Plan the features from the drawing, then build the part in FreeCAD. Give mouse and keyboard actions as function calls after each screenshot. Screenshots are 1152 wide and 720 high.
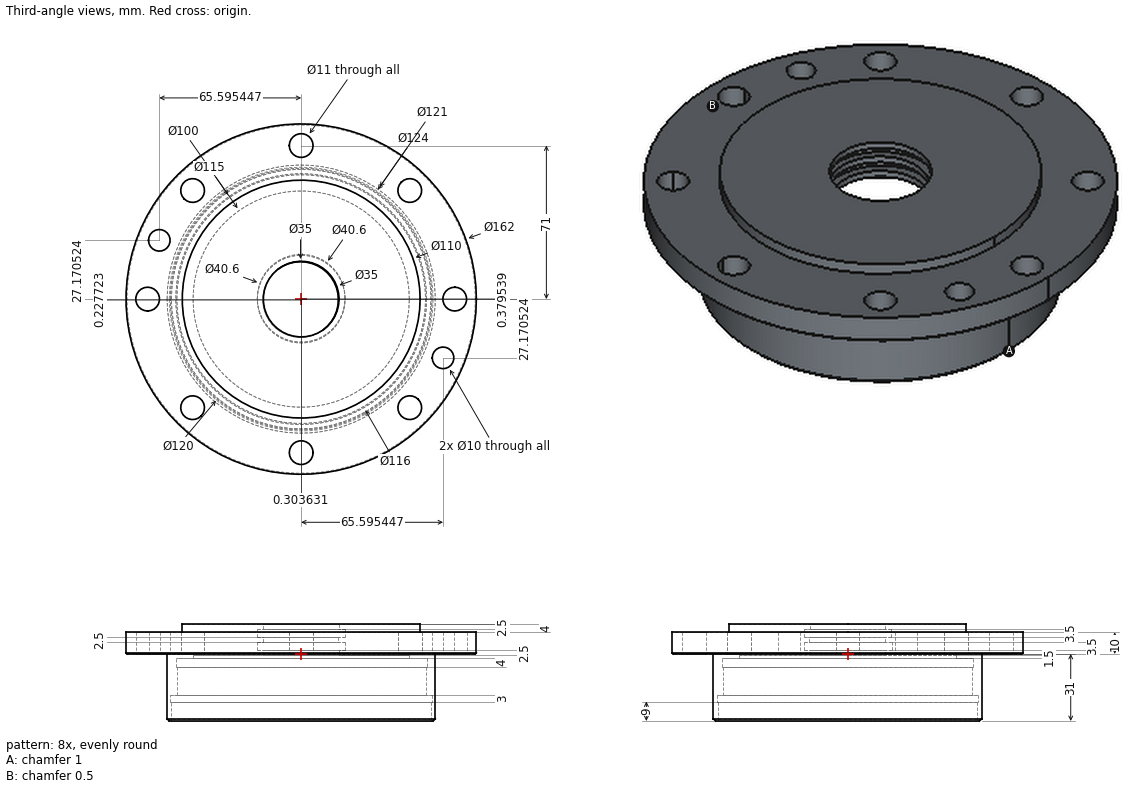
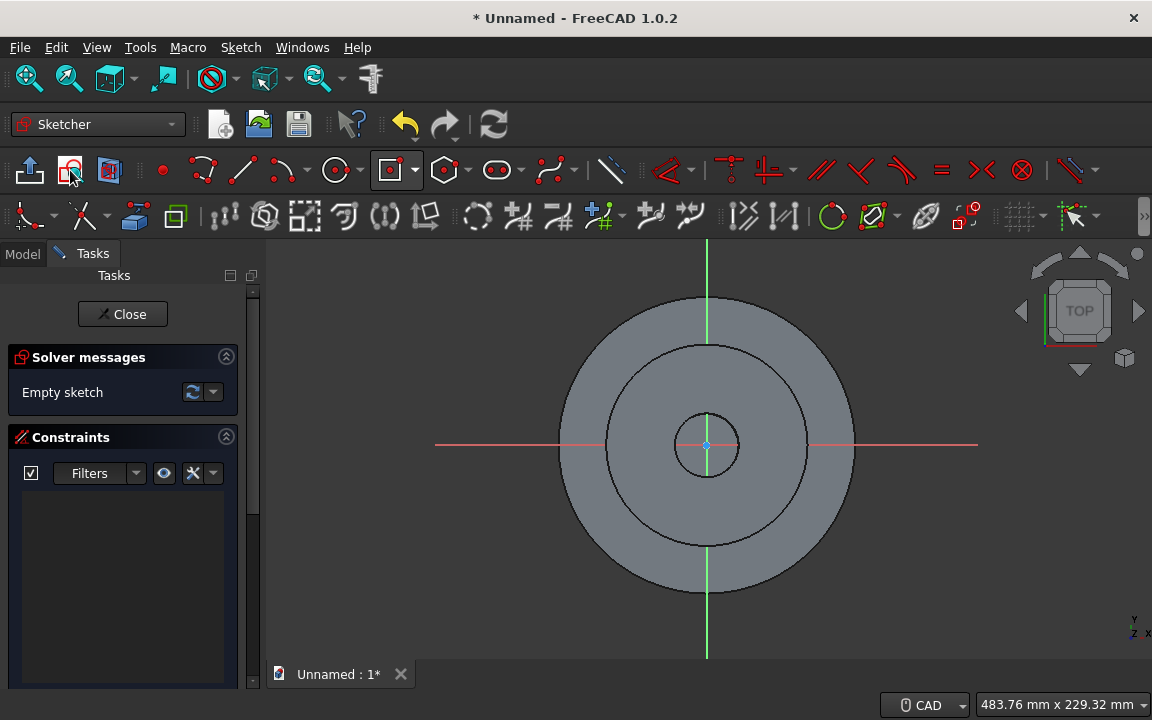
click(110, 170)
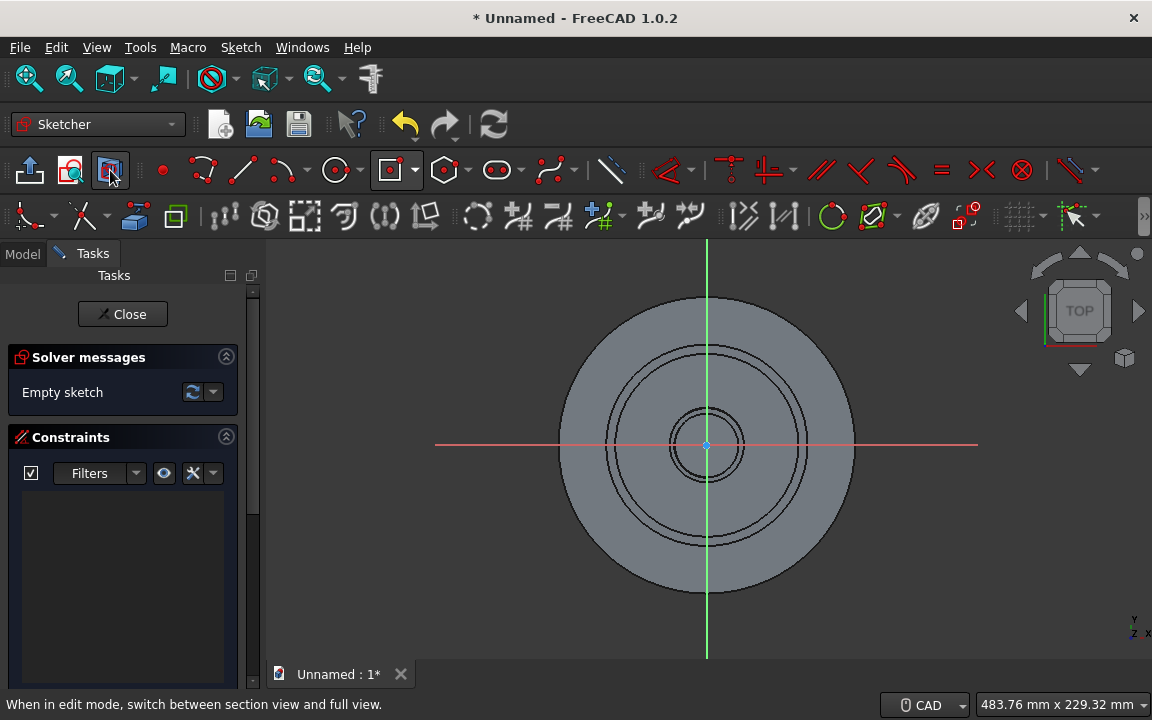
scroll(712, 305, up, 13)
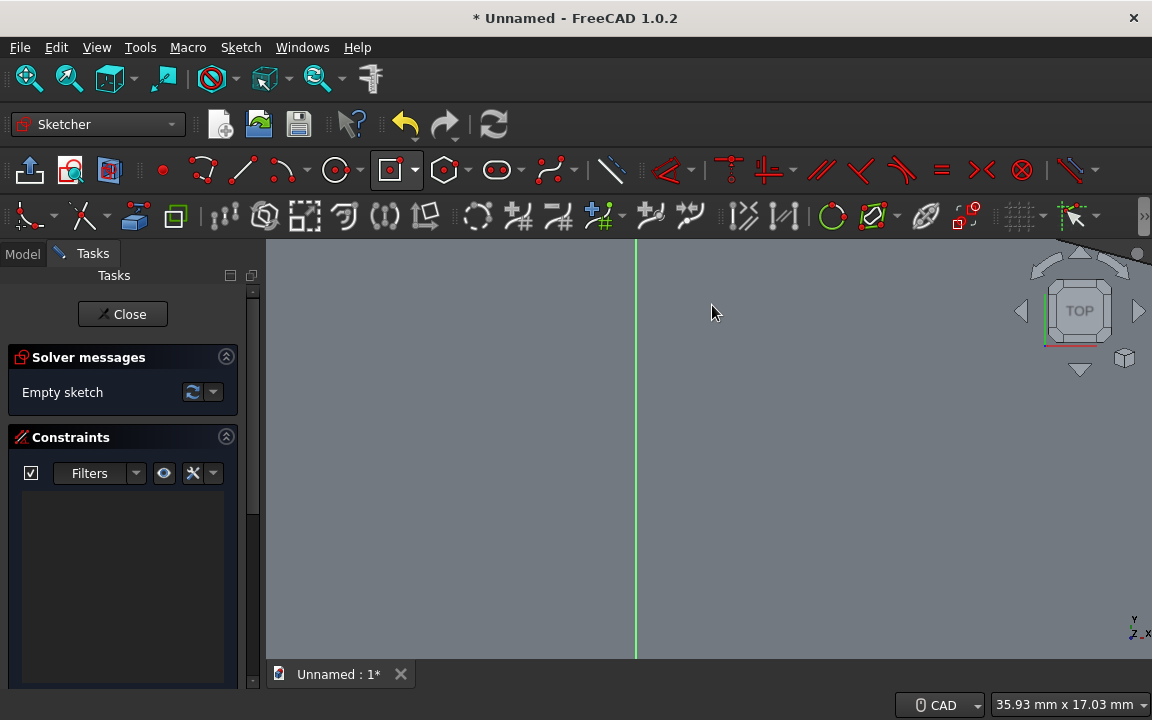
click(336, 170)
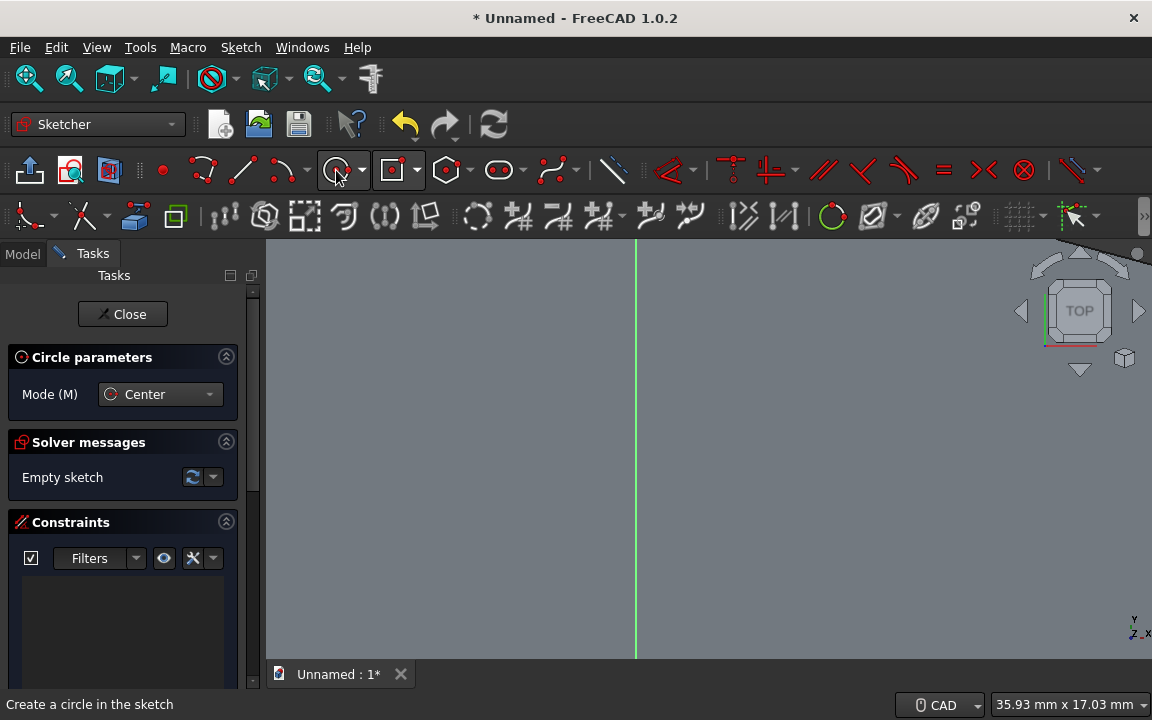
click(636, 441)
click(732, 345)
key(Escape)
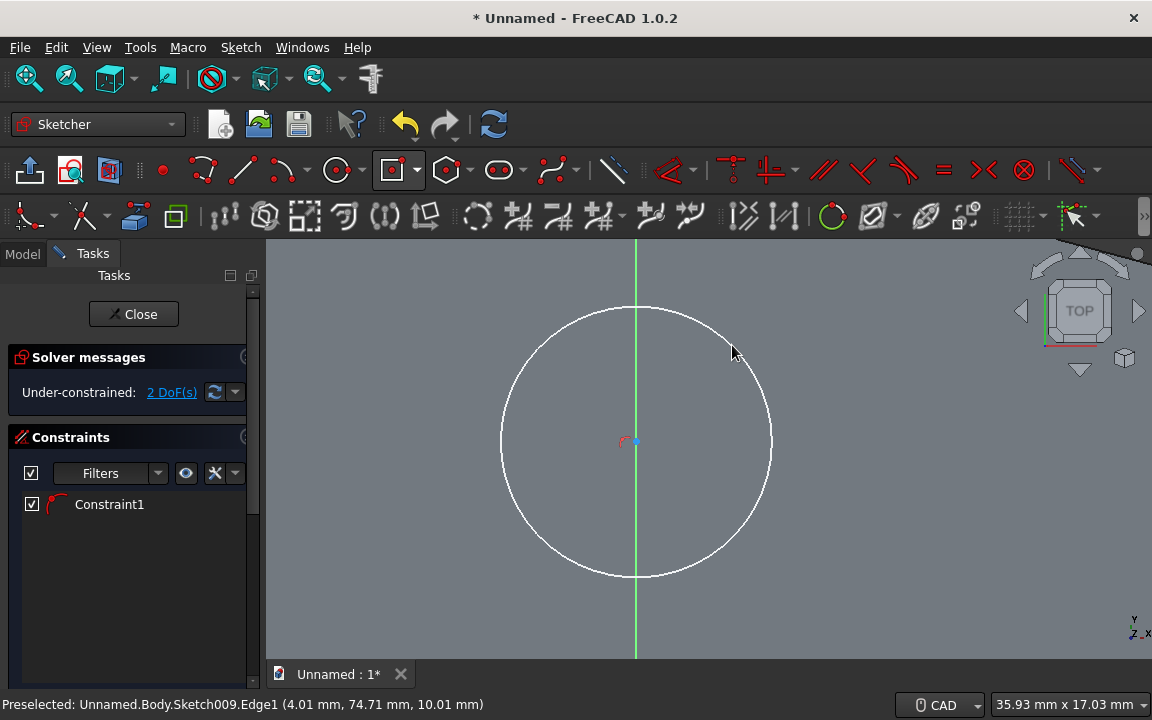
click(668, 170)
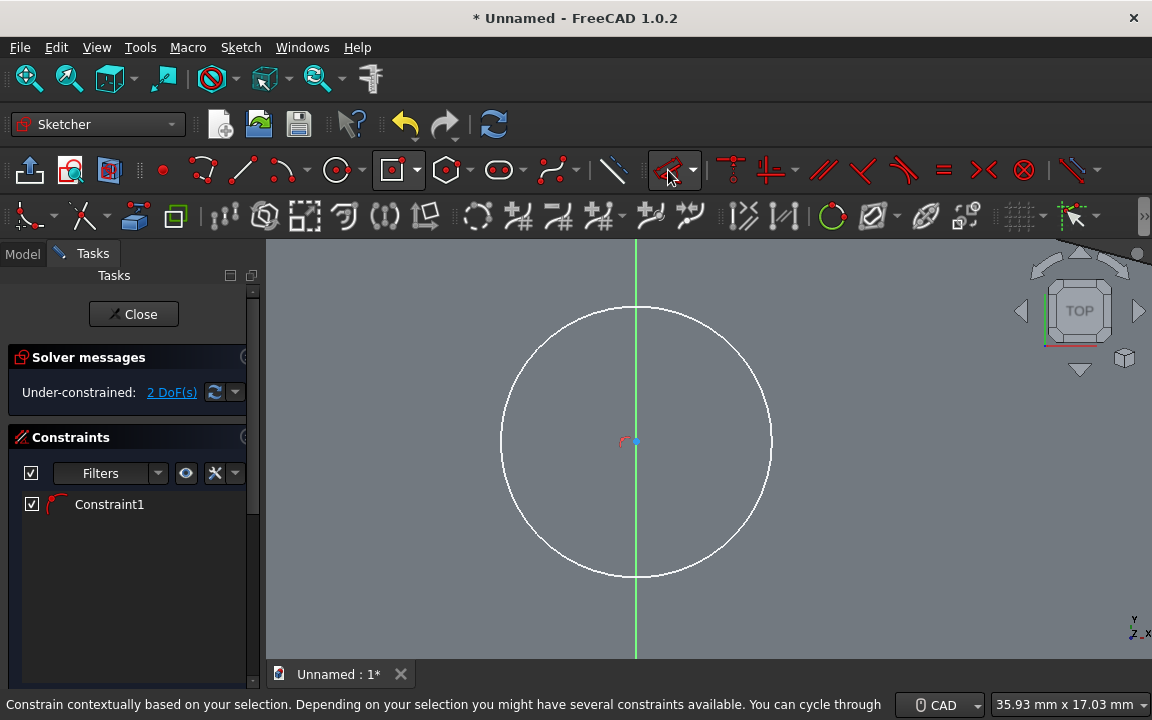
click(732, 346)
click(755, 323)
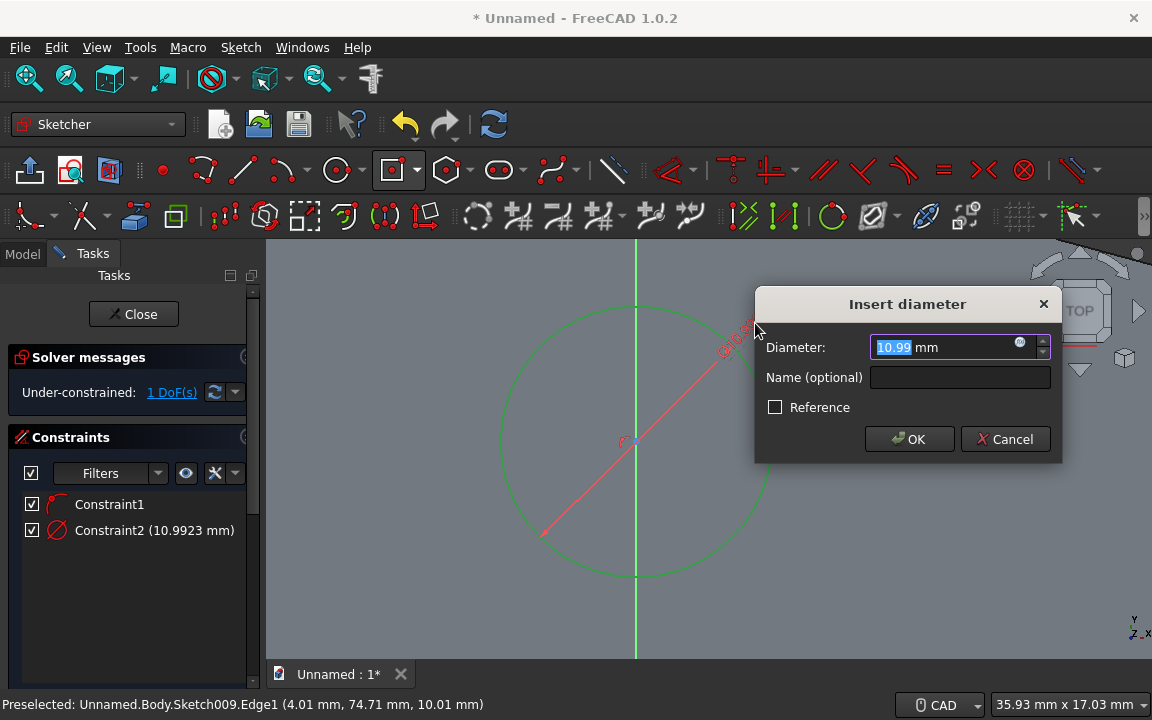
text(11)
key(Return)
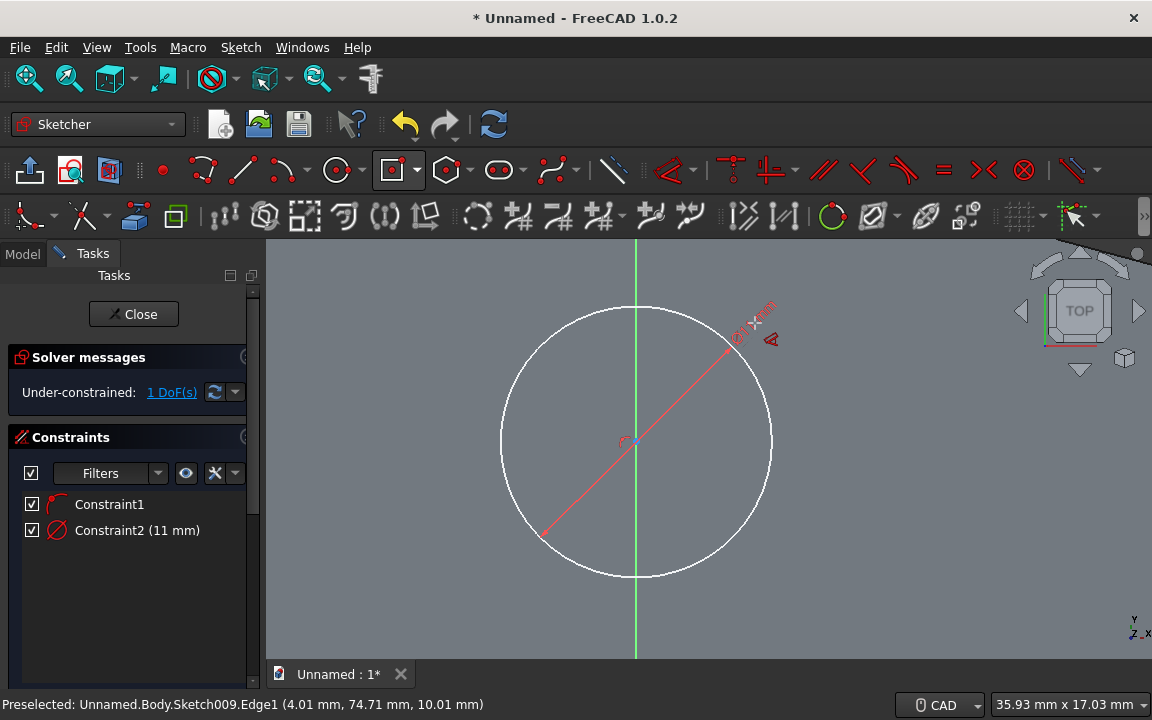
click(636, 442)
click(670, 537)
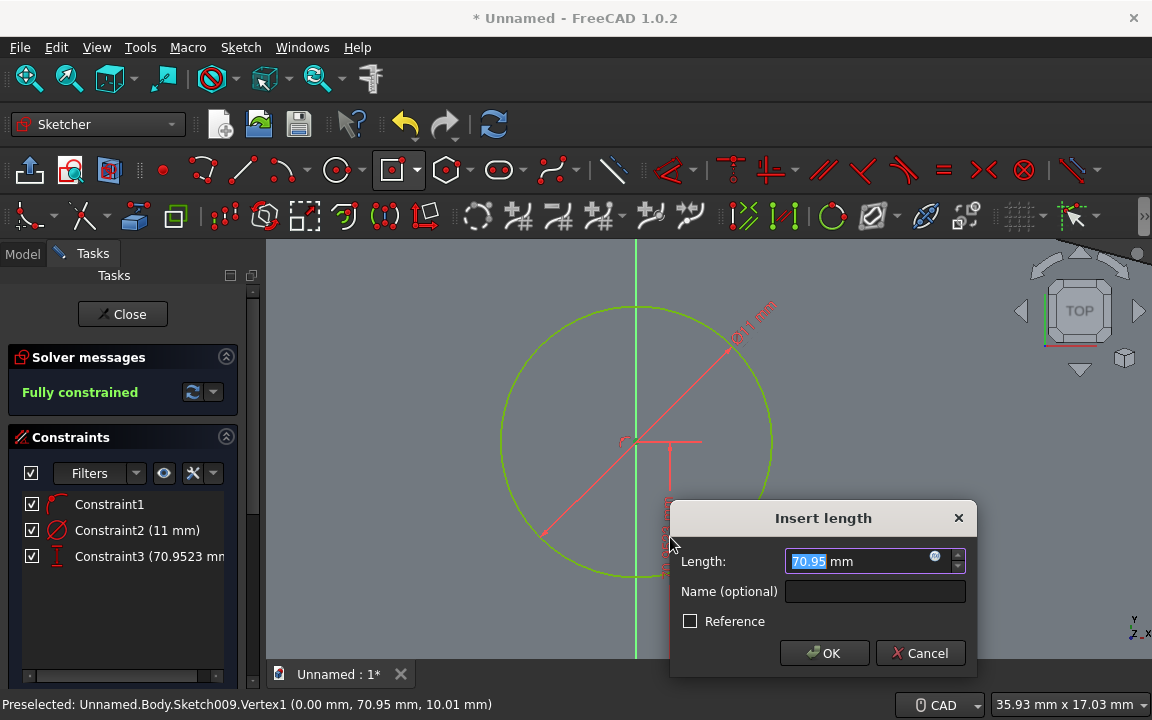
text(71)
key(Return)
key(Escape)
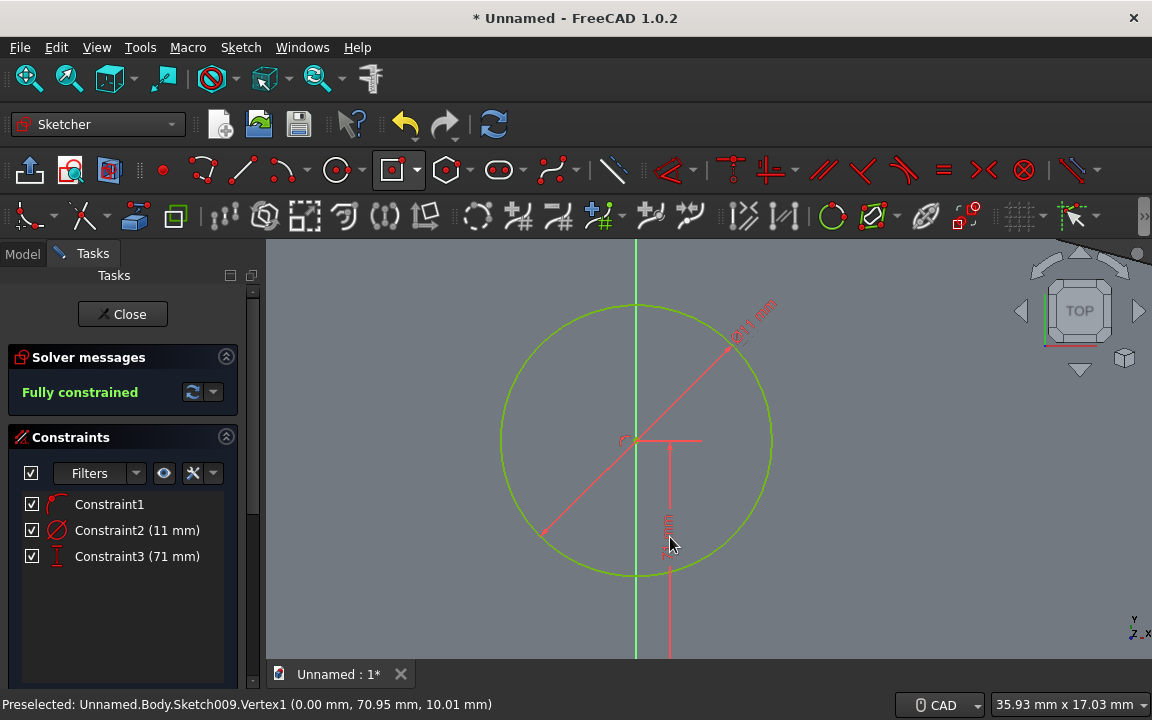
click(123, 314)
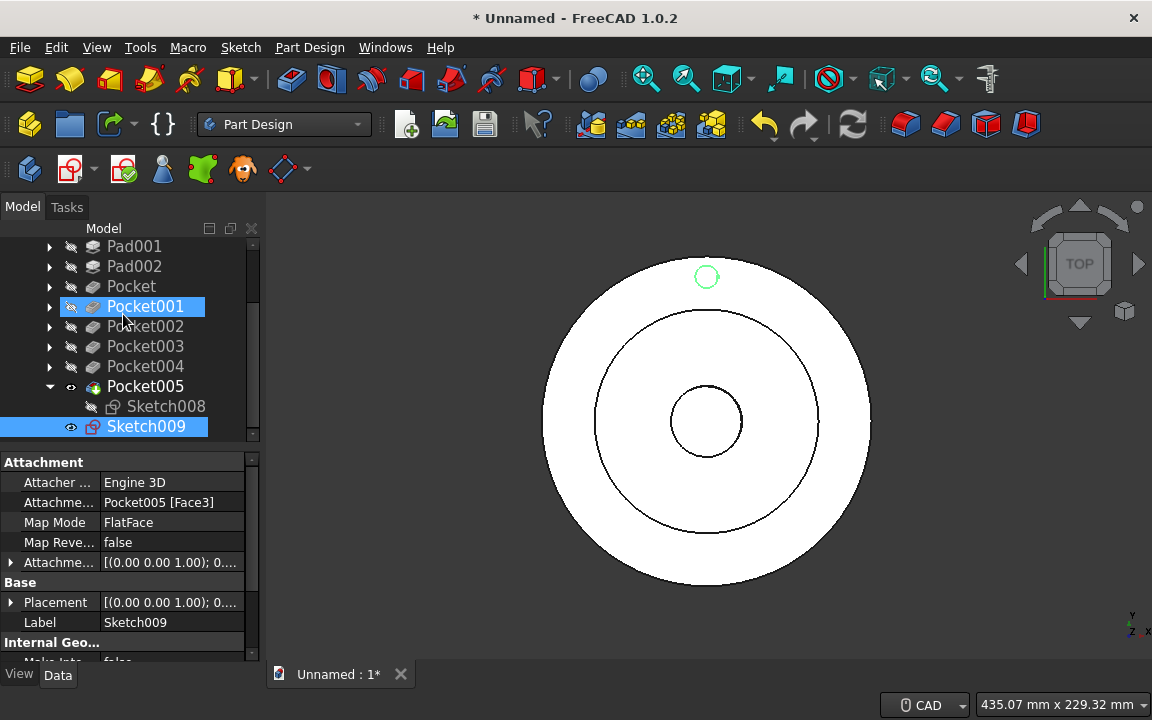
click(332, 80)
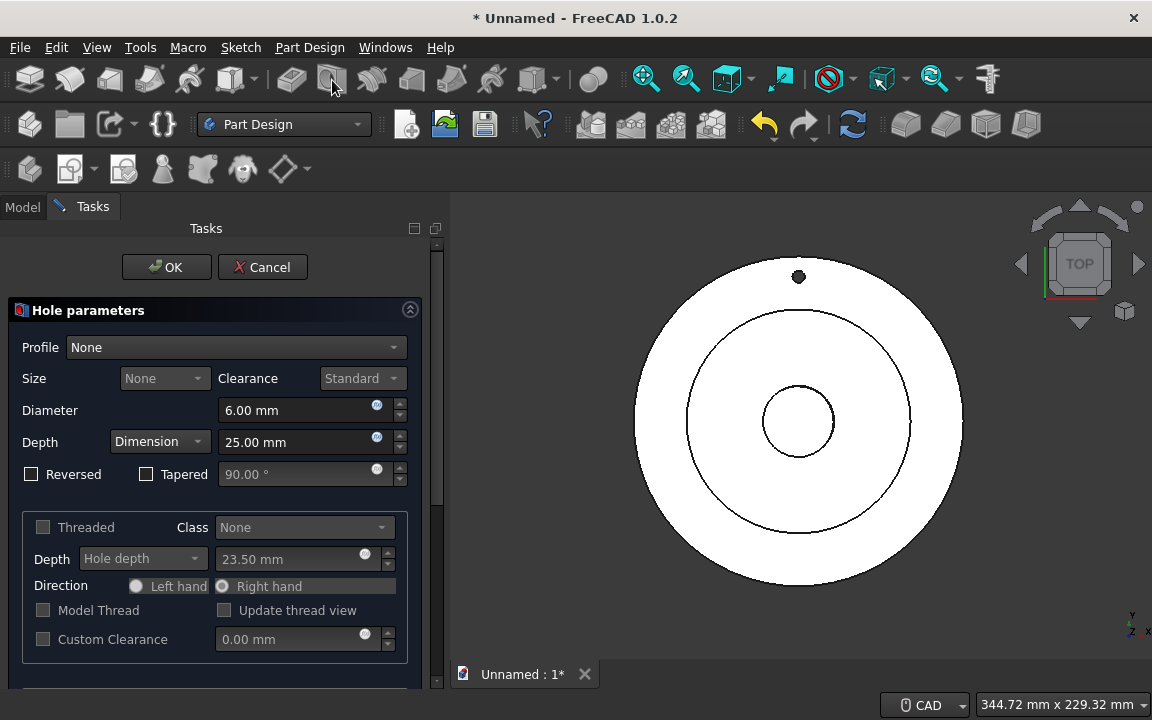
triple_click(305, 410)